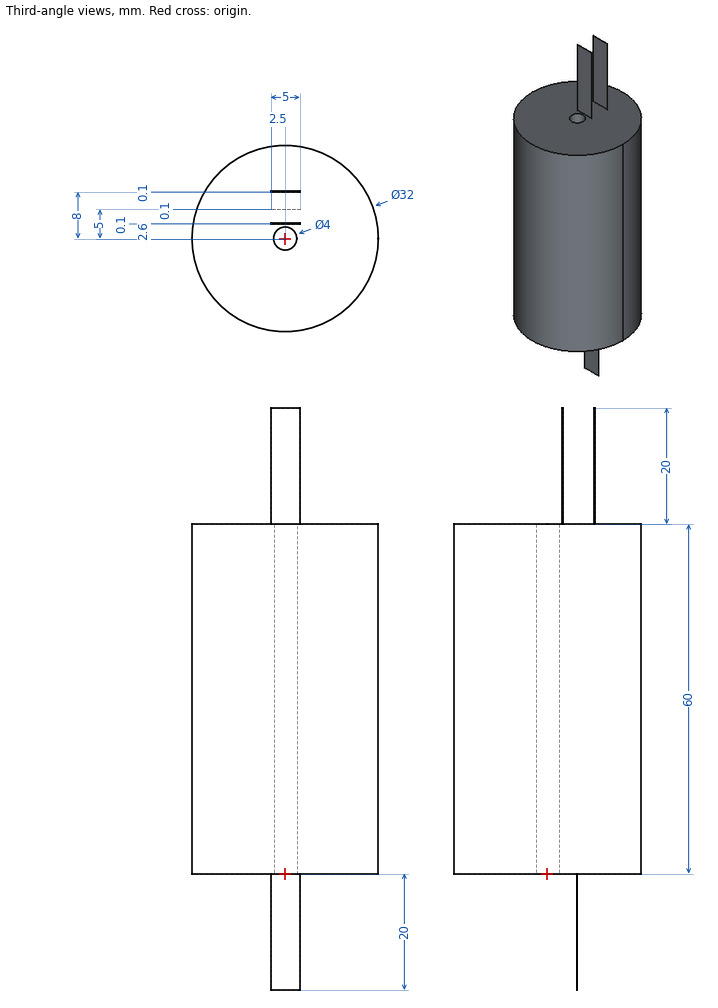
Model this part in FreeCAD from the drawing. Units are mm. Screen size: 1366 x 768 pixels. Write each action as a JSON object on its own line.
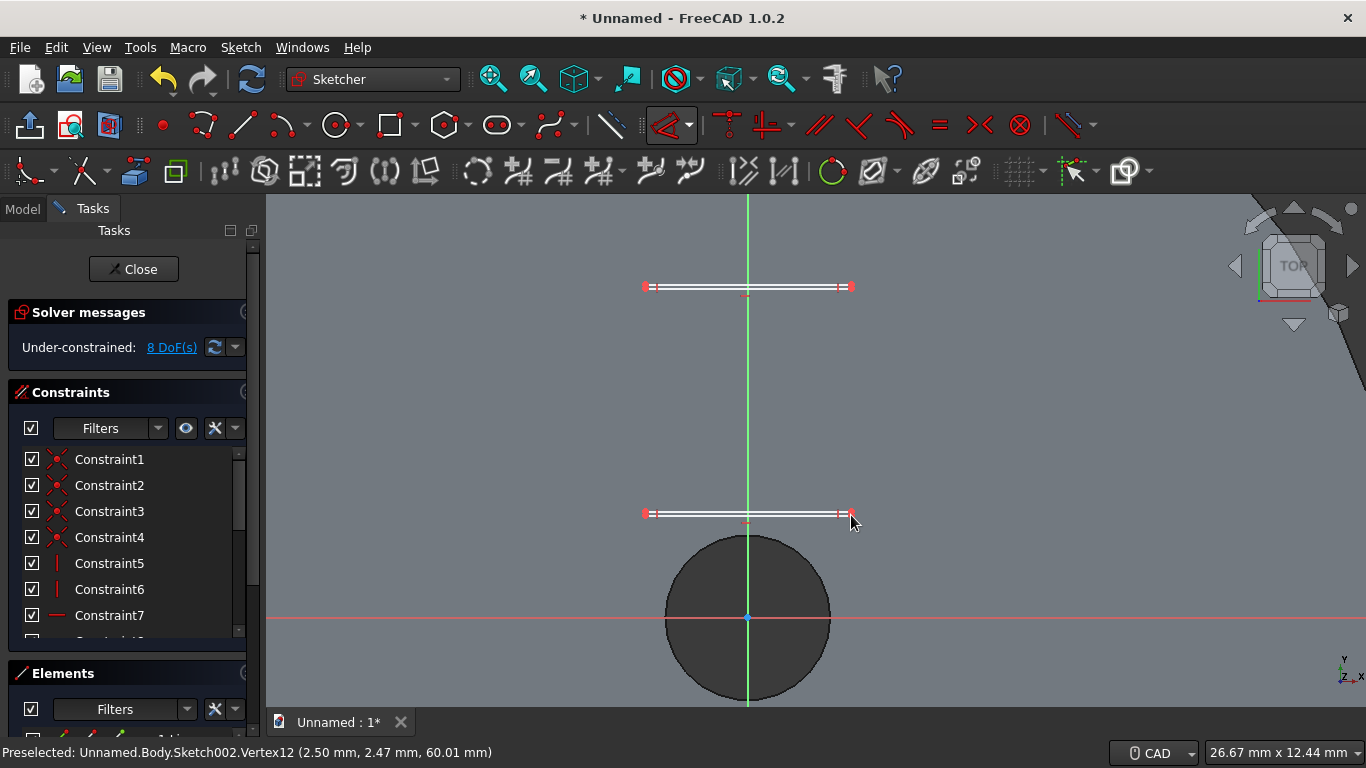
{"action": "scroll", "coordinate": [707, 289], "scroll_direction": "up", "scroll_amount": 7}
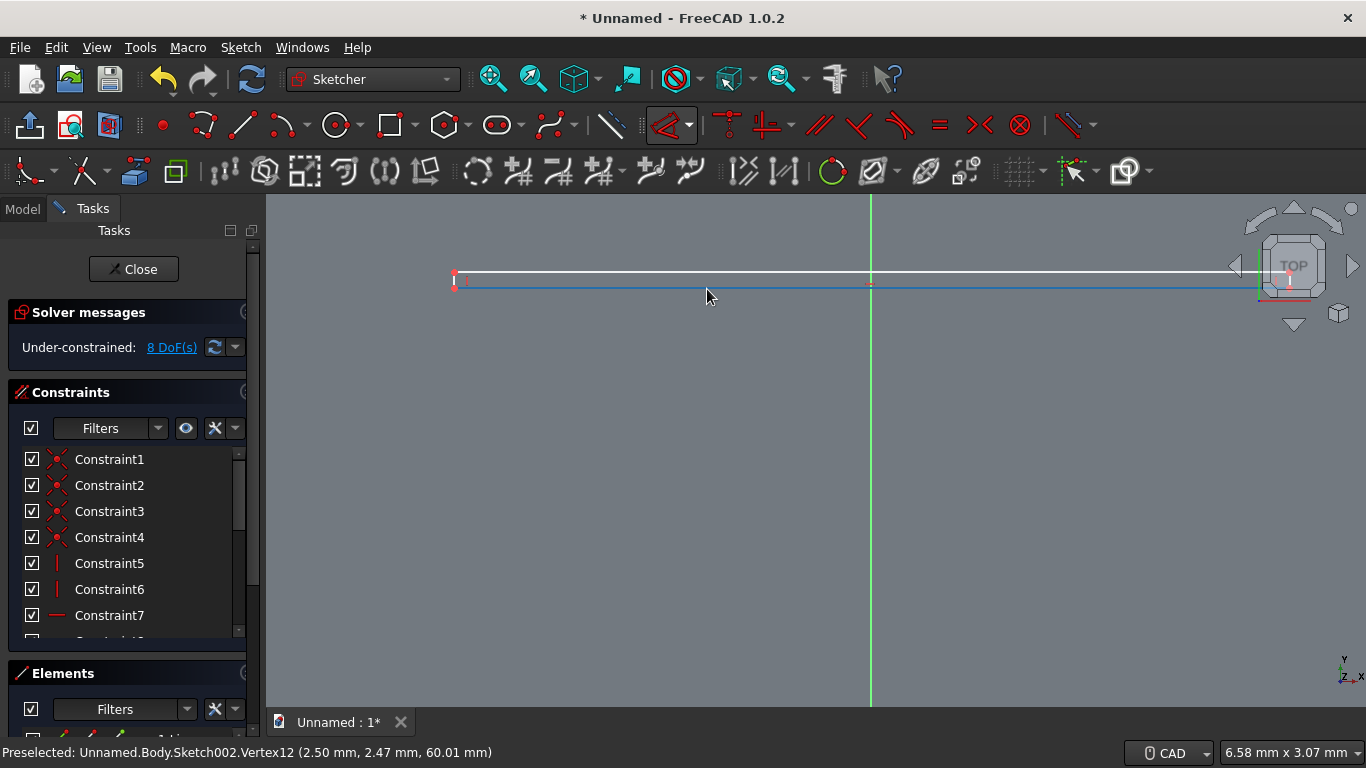
{"action": "left_click", "coordinate": [705, 288]}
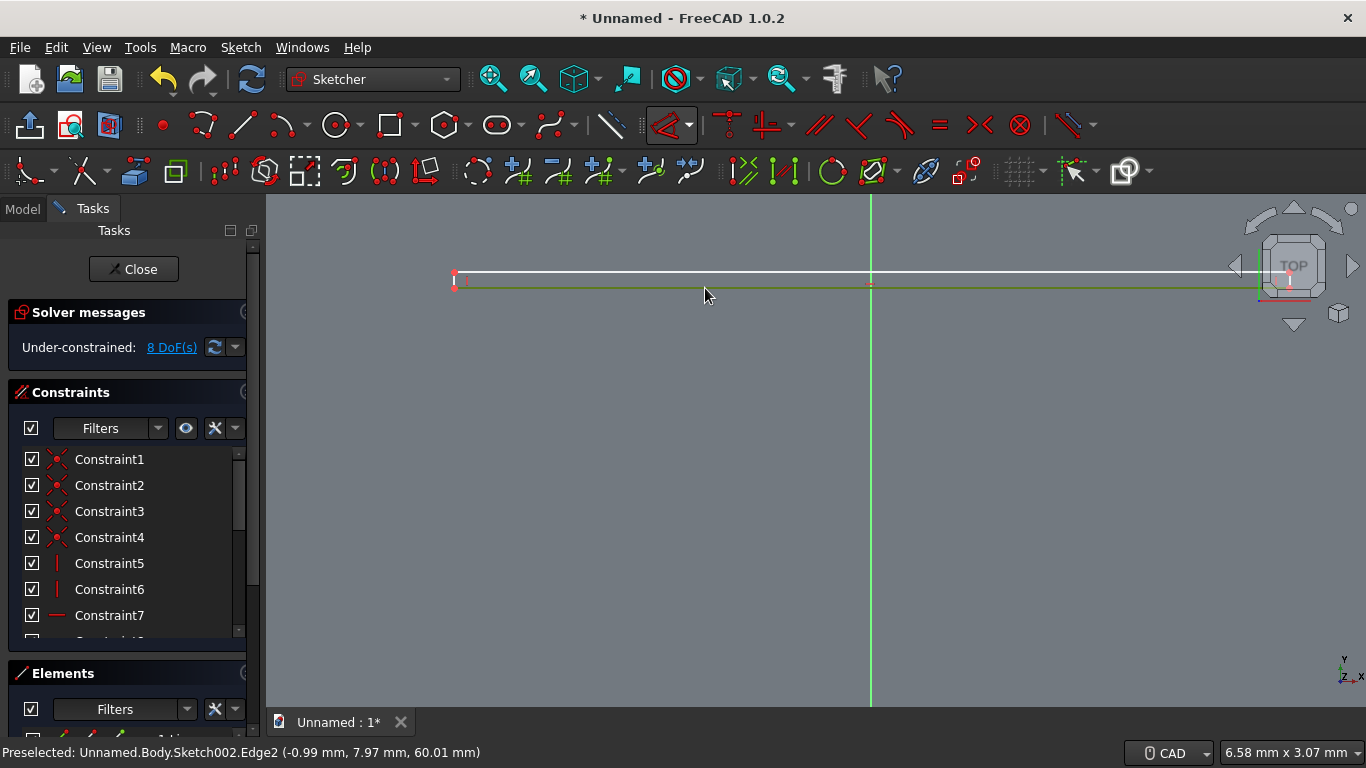
{"action": "left_click", "coordinate": [692, 126]}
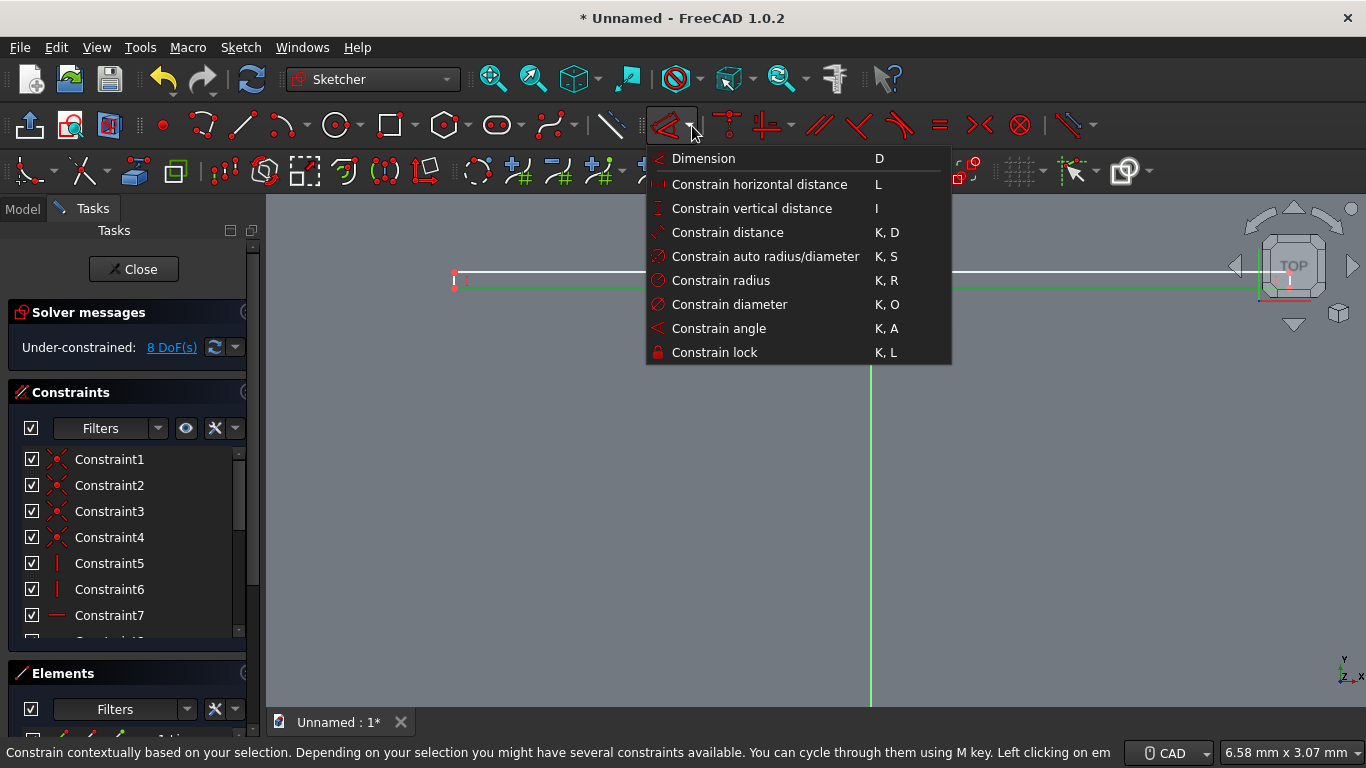
{"action": "left_click", "coordinate": [799, 184]}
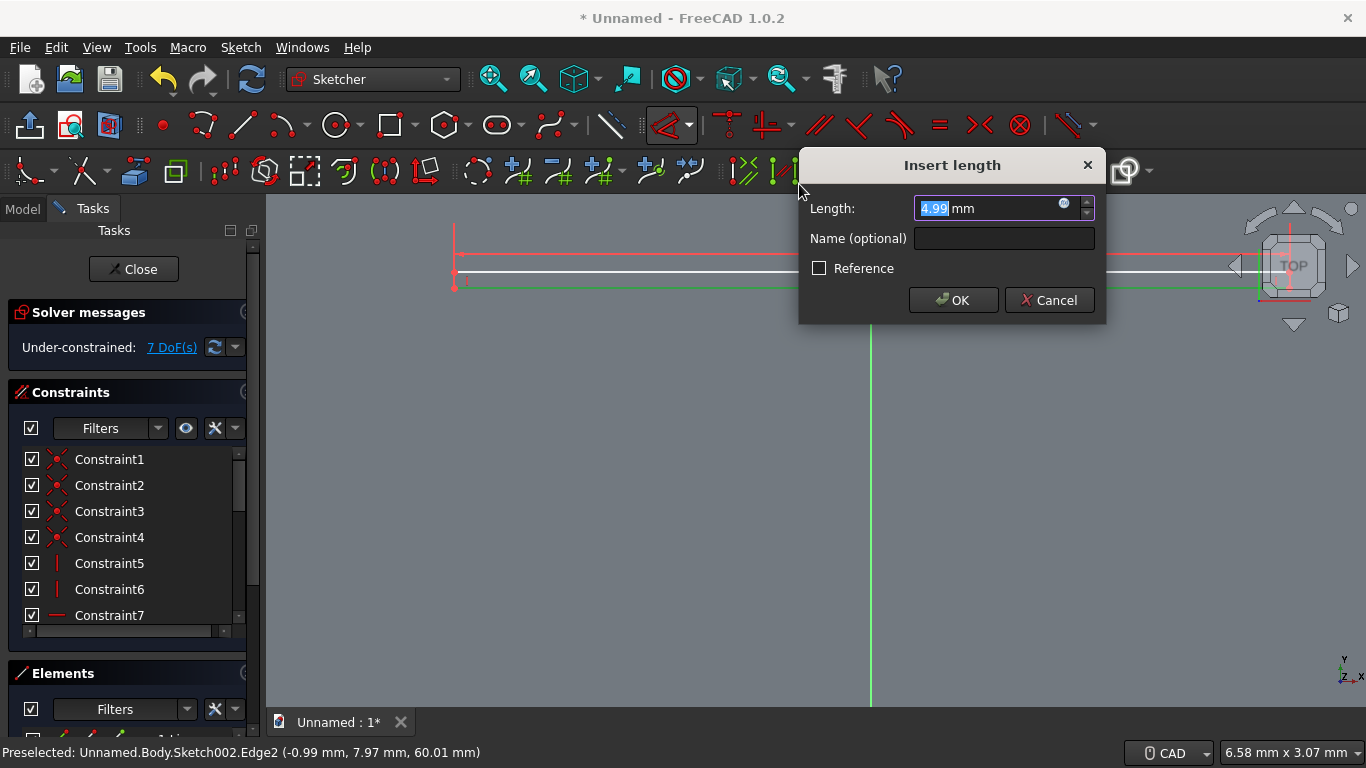
{"action": "type", "text": "5"}
{"action": "key", "text": "Return"}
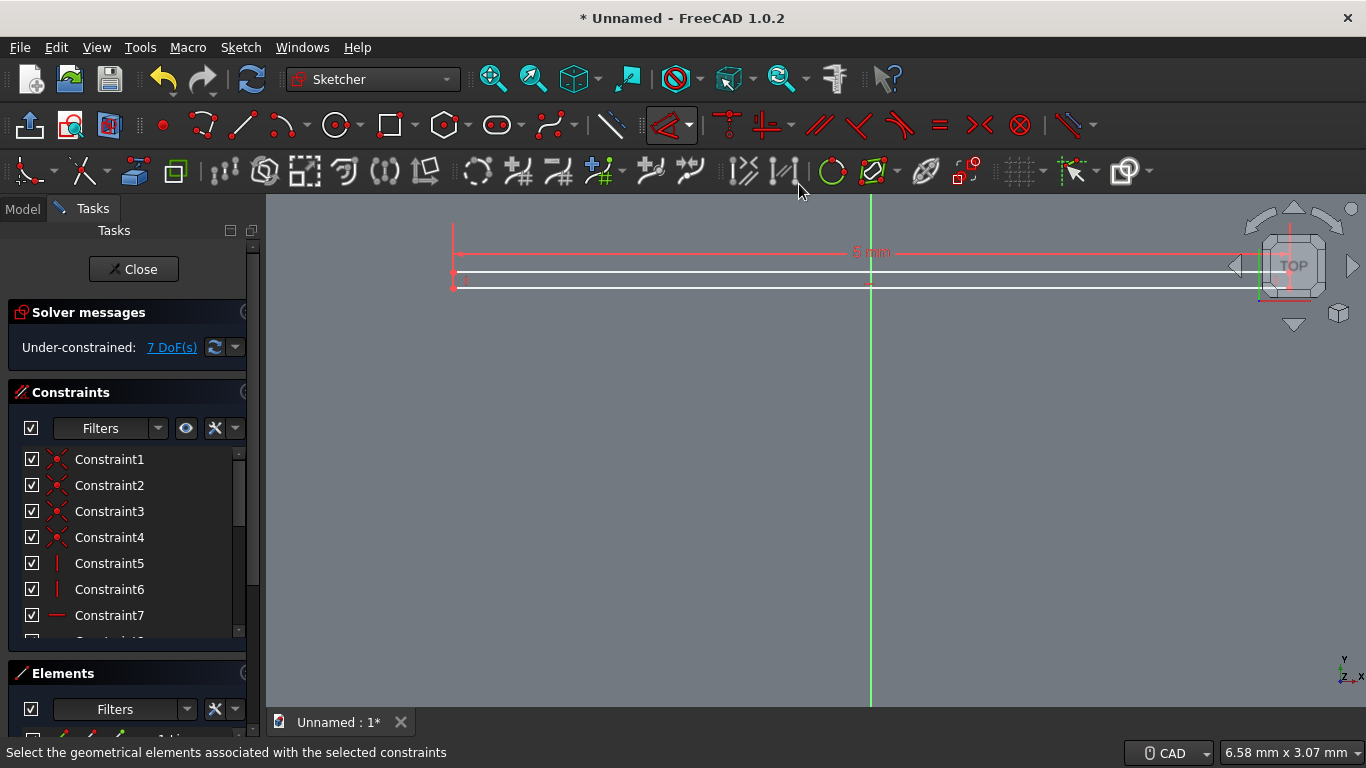
{"action": "scroll", "coordinate": [707, 289], "scroll_direction": "down", "scroll_amount": 7}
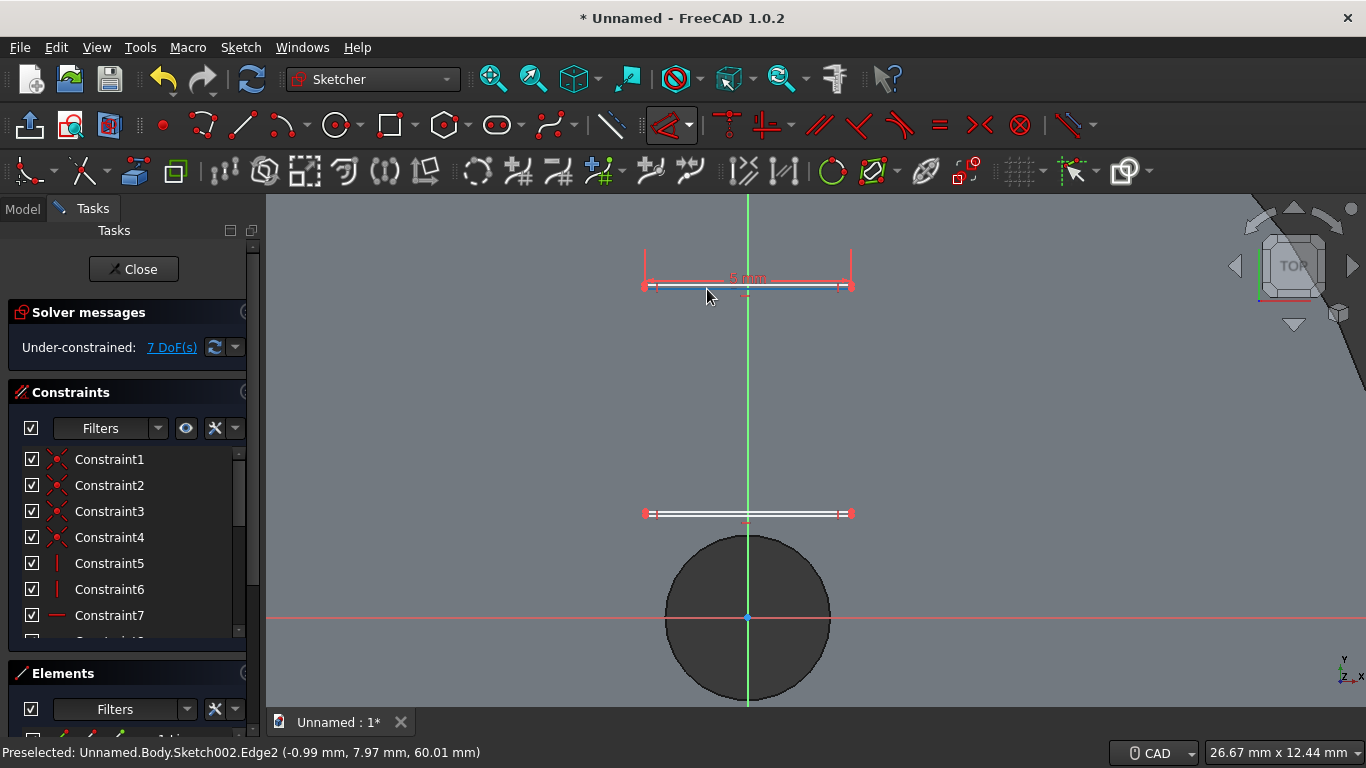
{"action": "scroll", "coordinate": [707, 516], "scroll_direction": "up", "scroll_amount": 7}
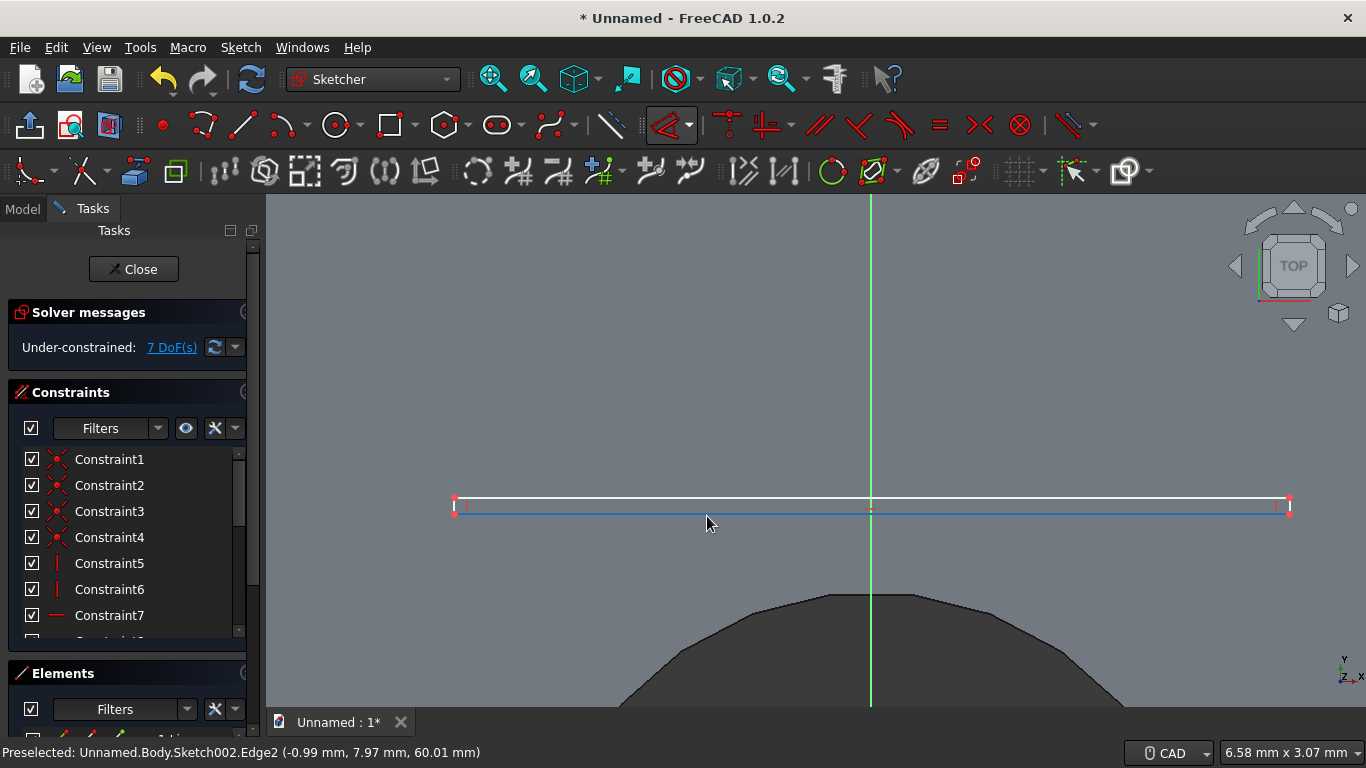
{"action": "left_click", "coordinate": [705, 514]}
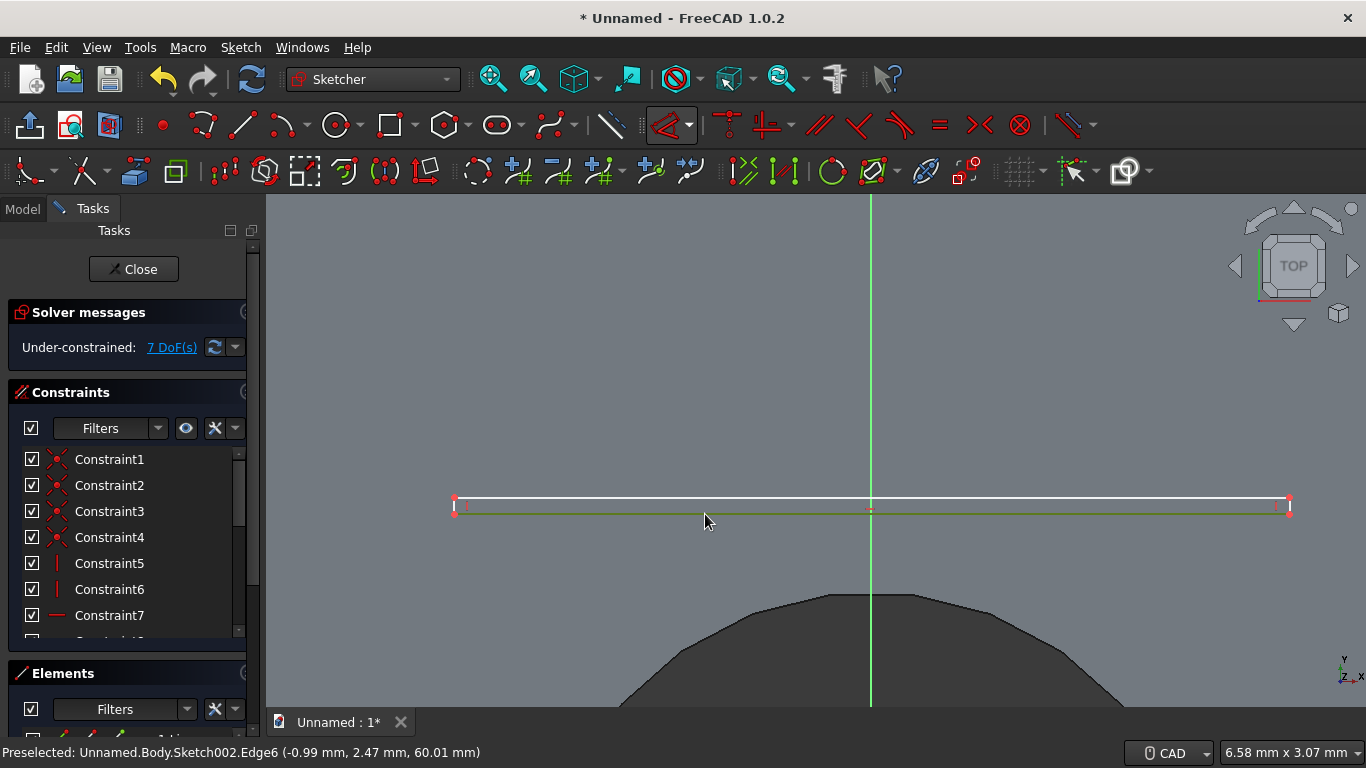
{"action": "left_click", "coordinate": [692, 126]}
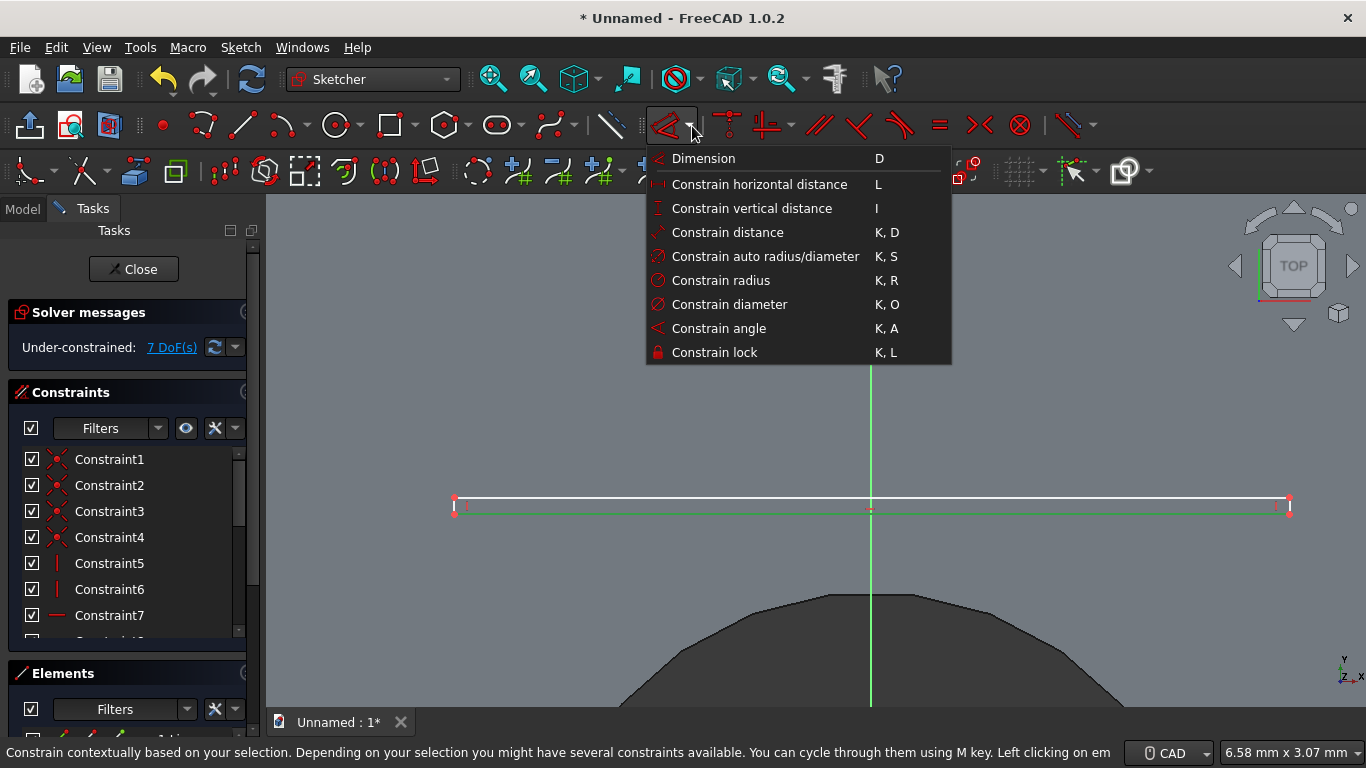
{"action": "left_click", "coordinate": [799, 184]}